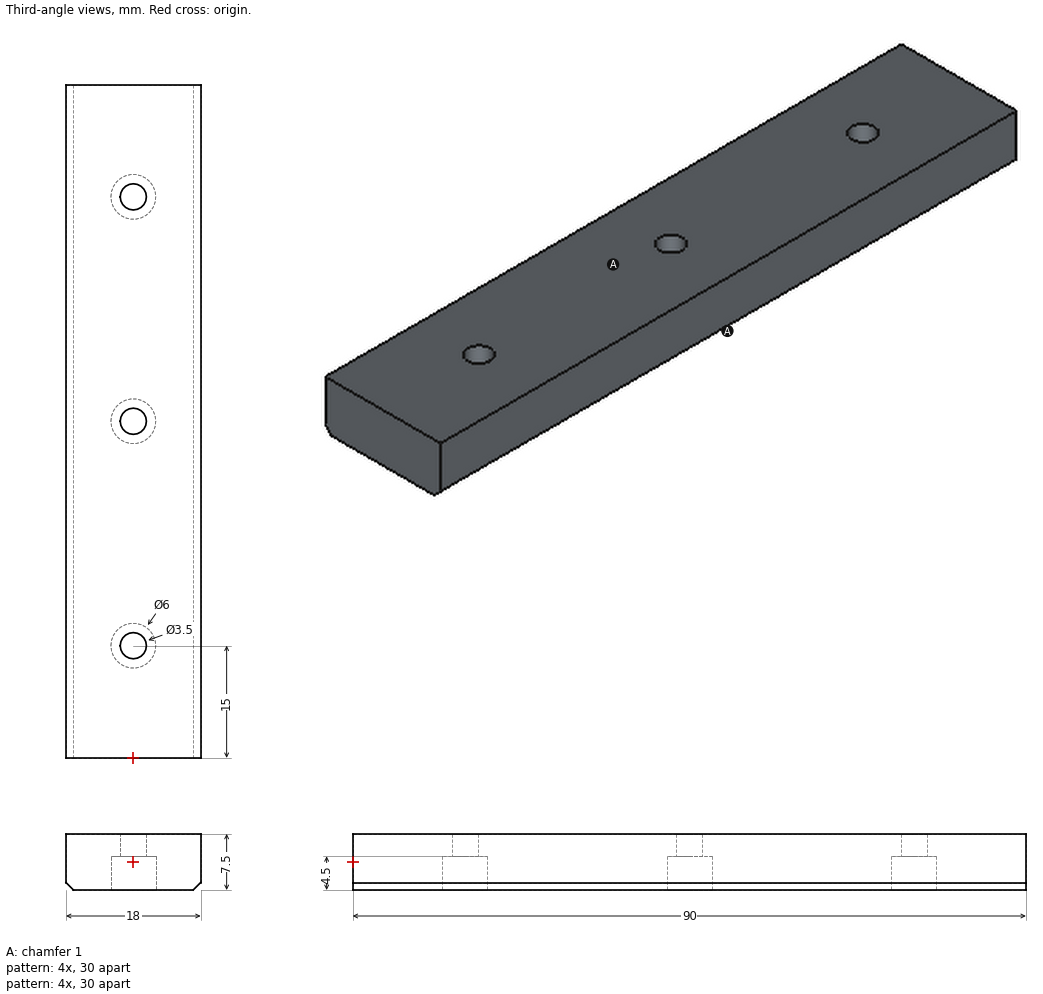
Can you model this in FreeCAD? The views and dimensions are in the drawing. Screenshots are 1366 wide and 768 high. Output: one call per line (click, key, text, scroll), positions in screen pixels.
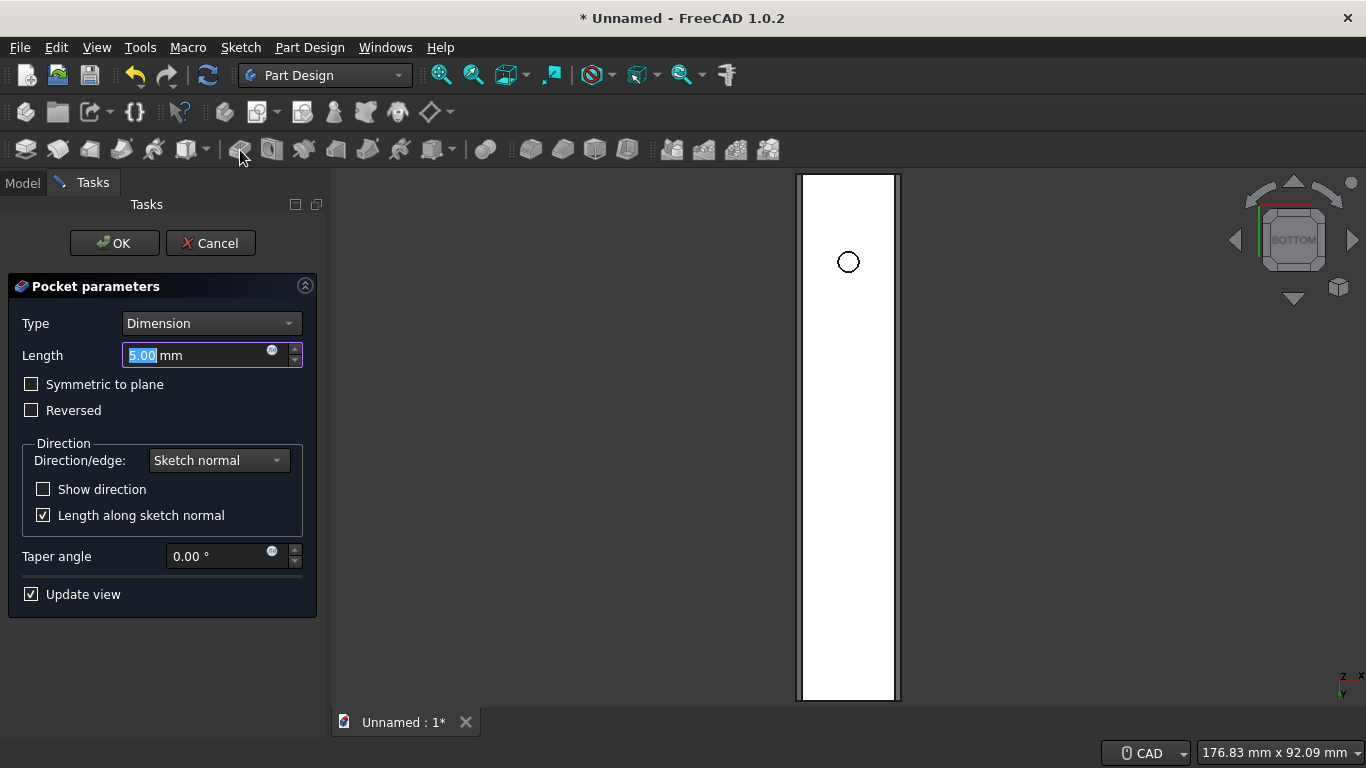
click(212, 324)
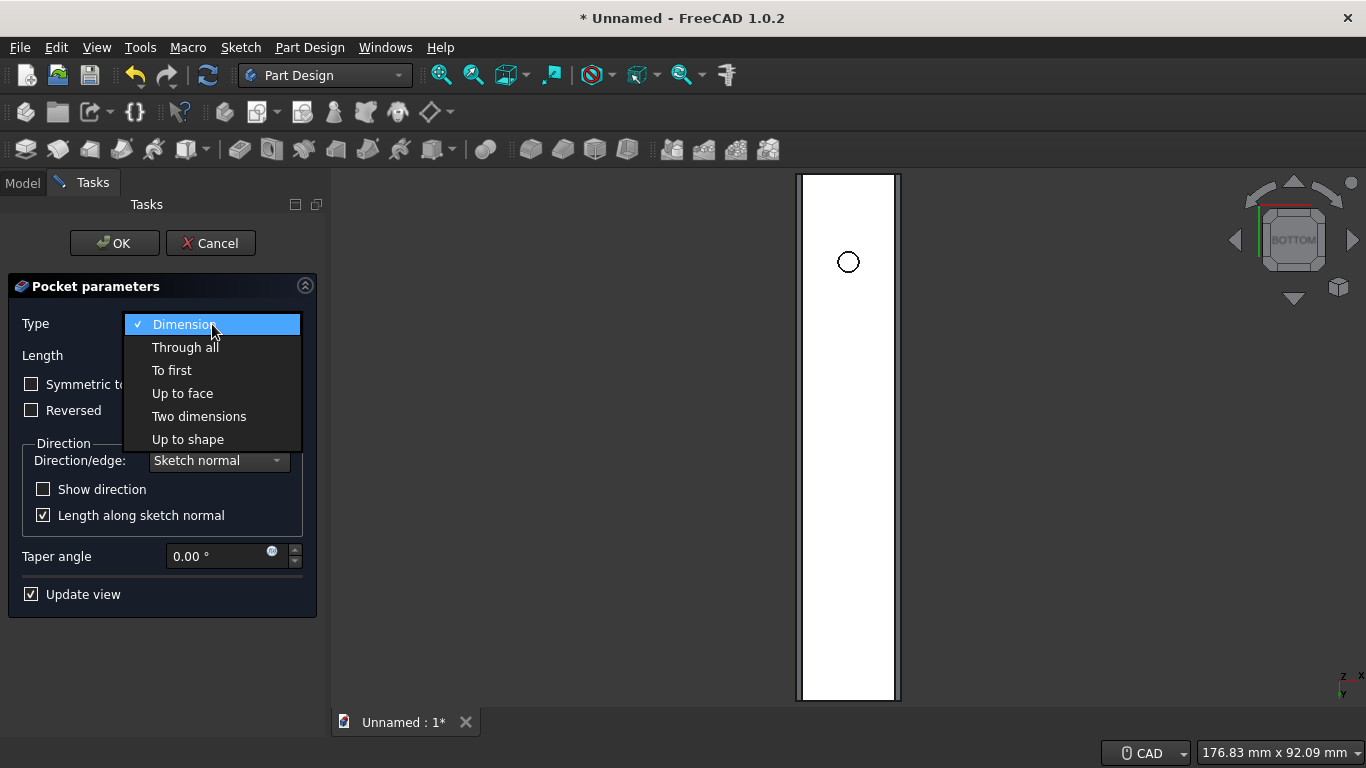
click(212, 348)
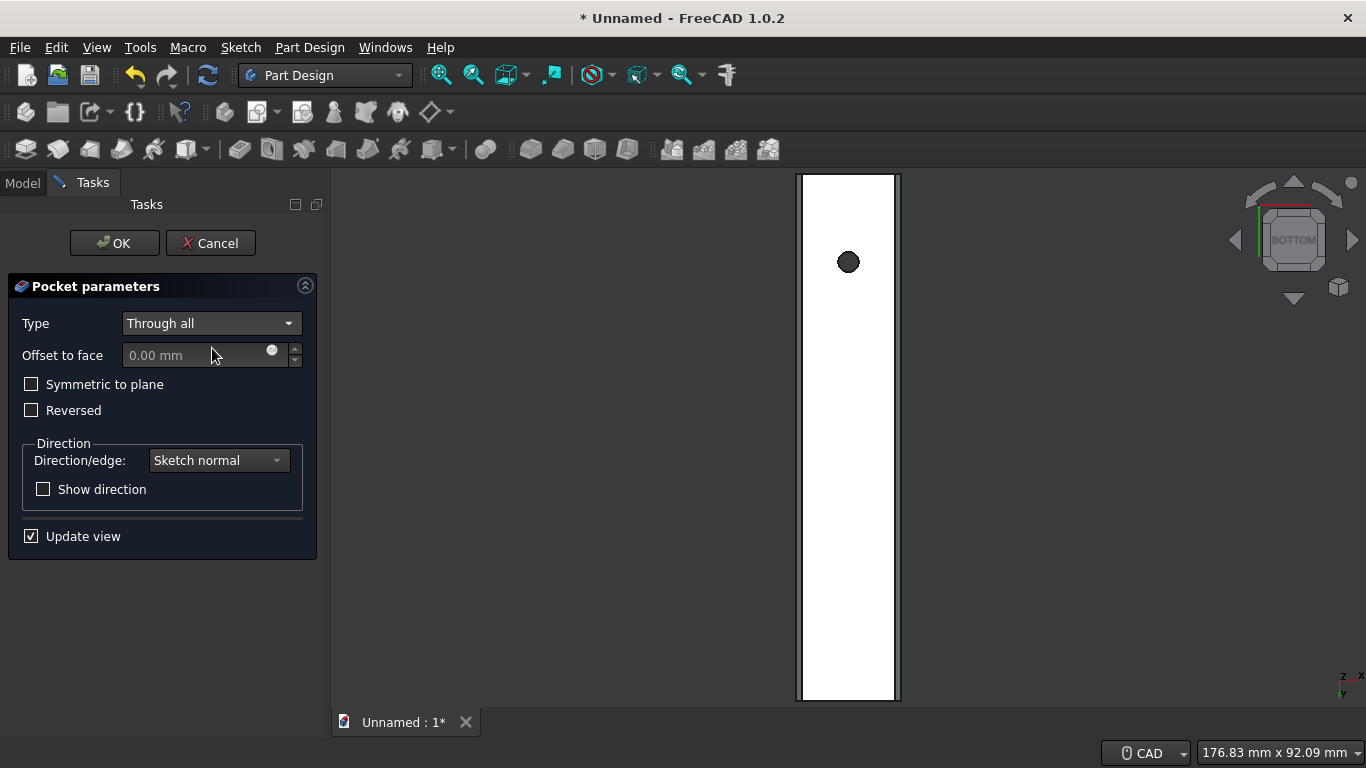
click(115, 243)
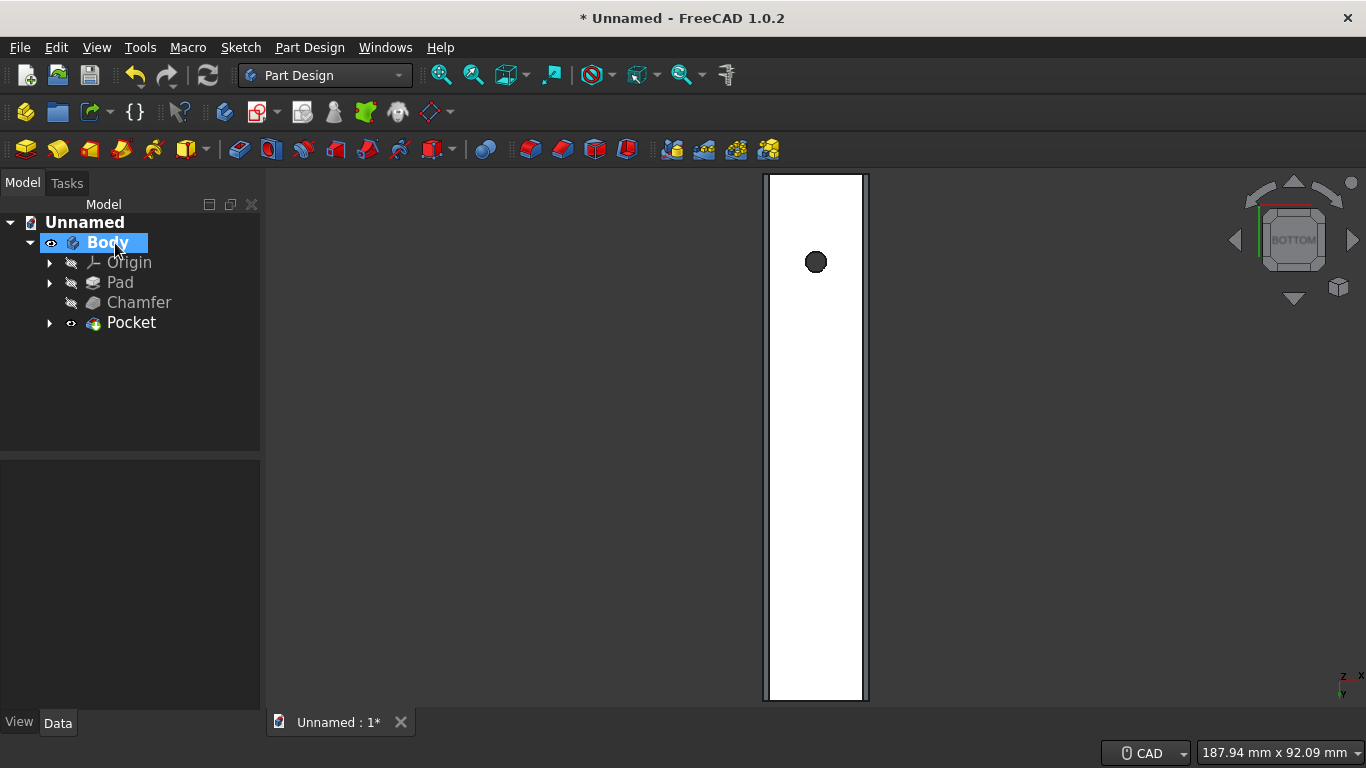
click(816, 587)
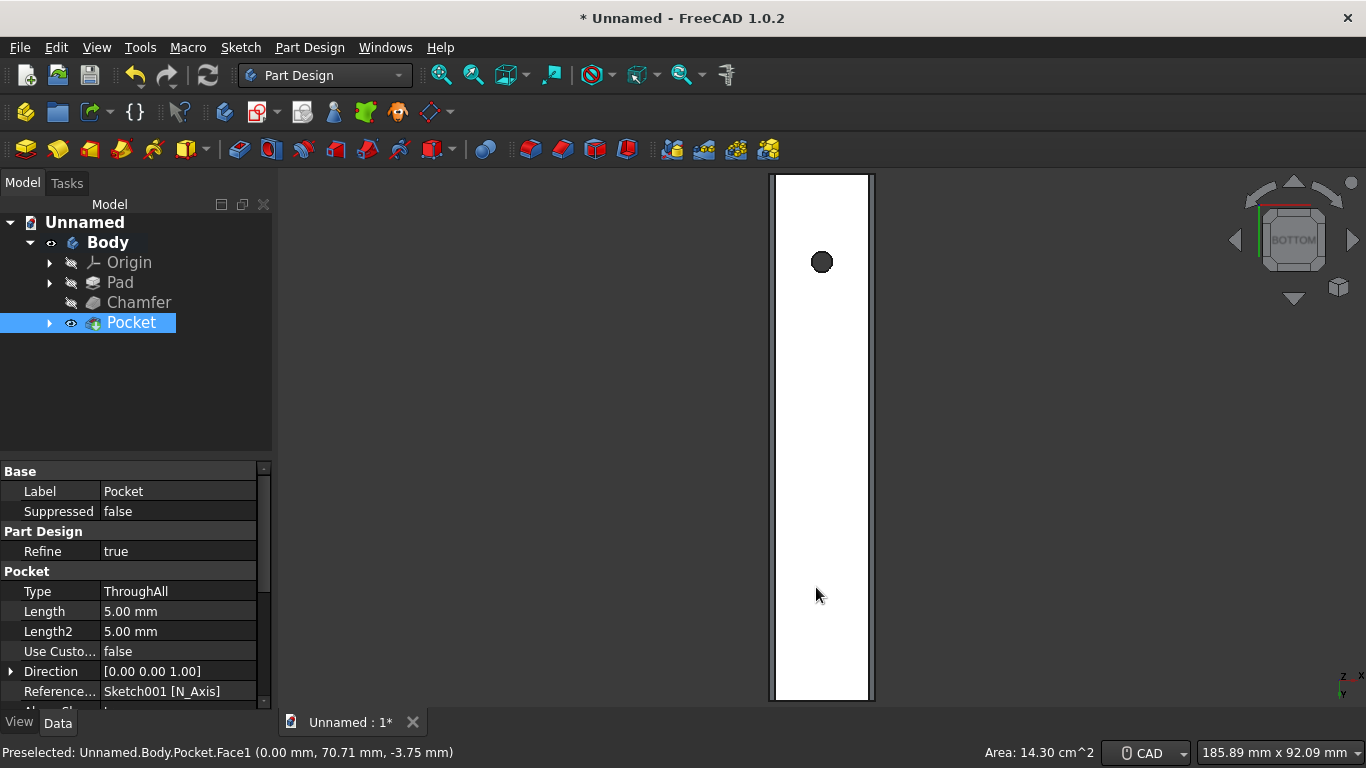
click(258, 112)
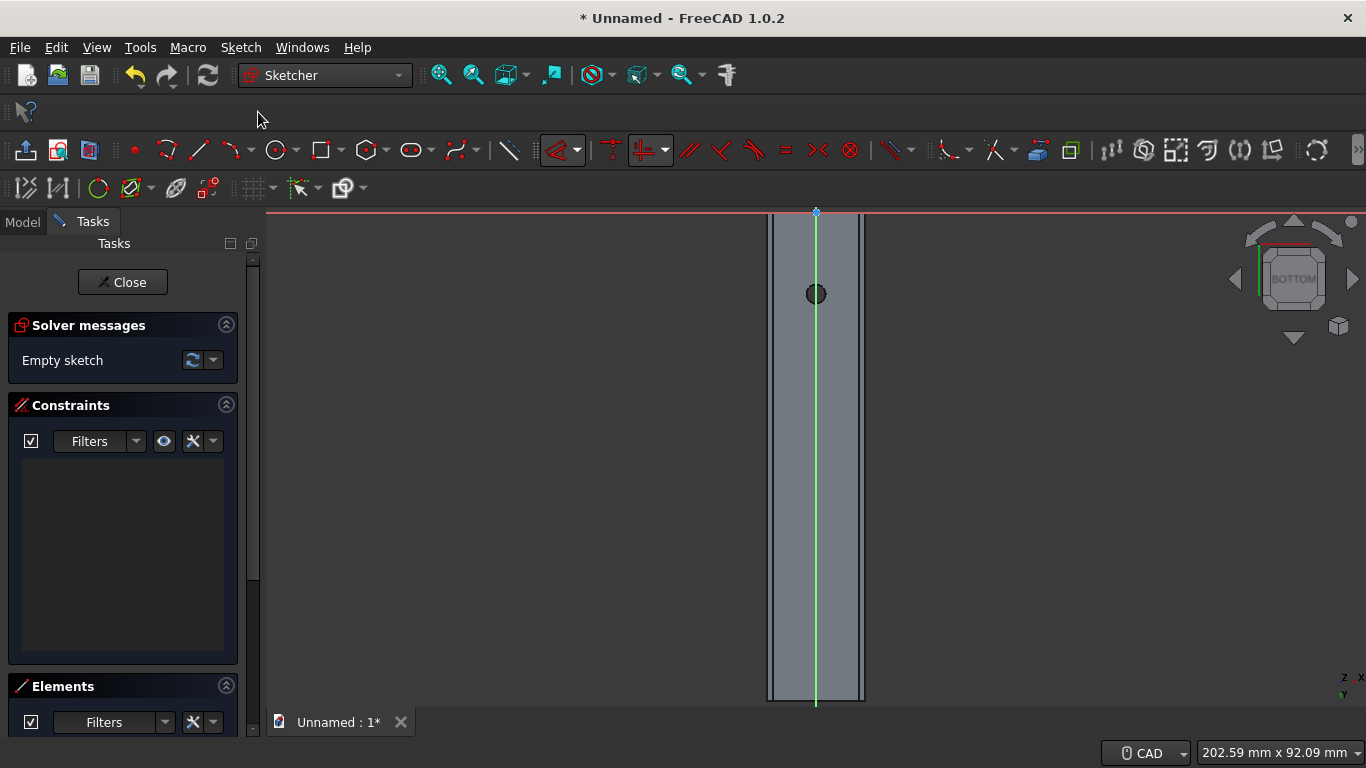
scroll(825, 274, up, 11)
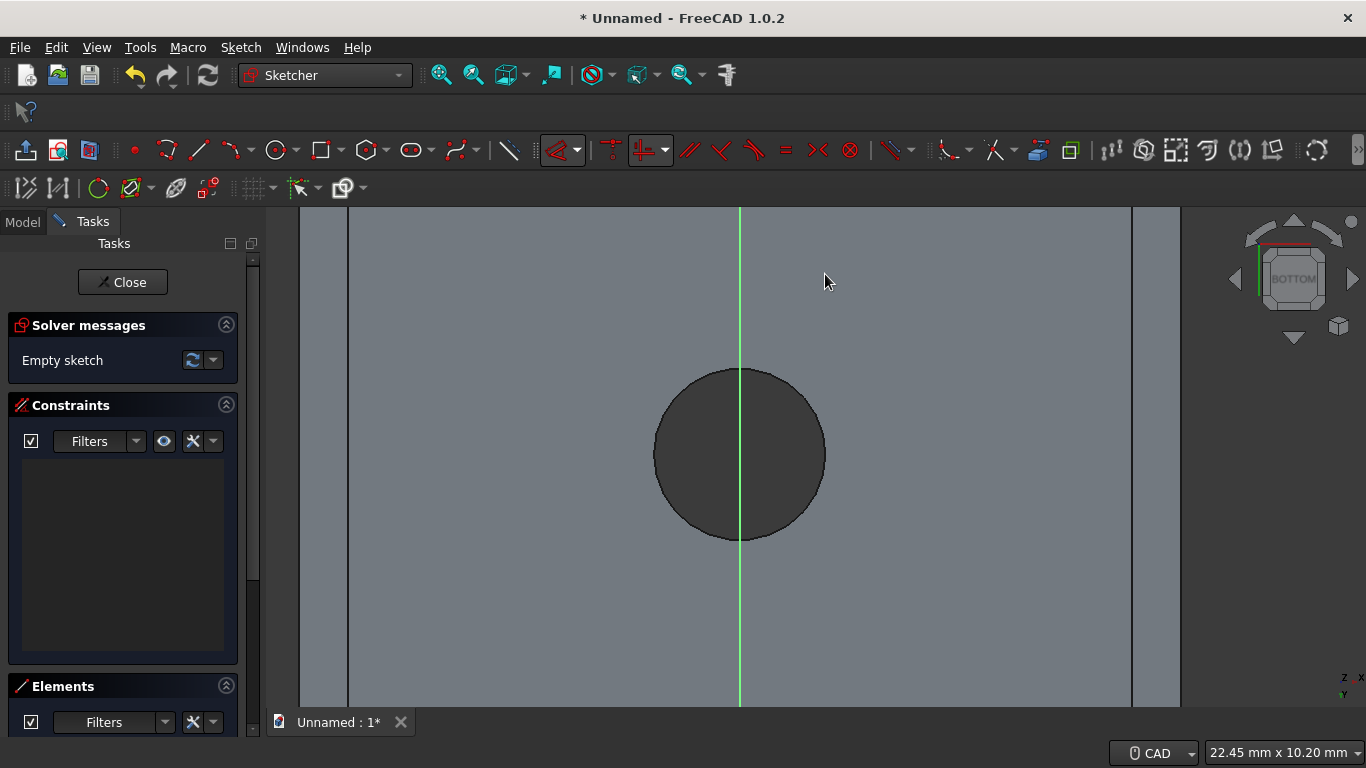
click(276, 150)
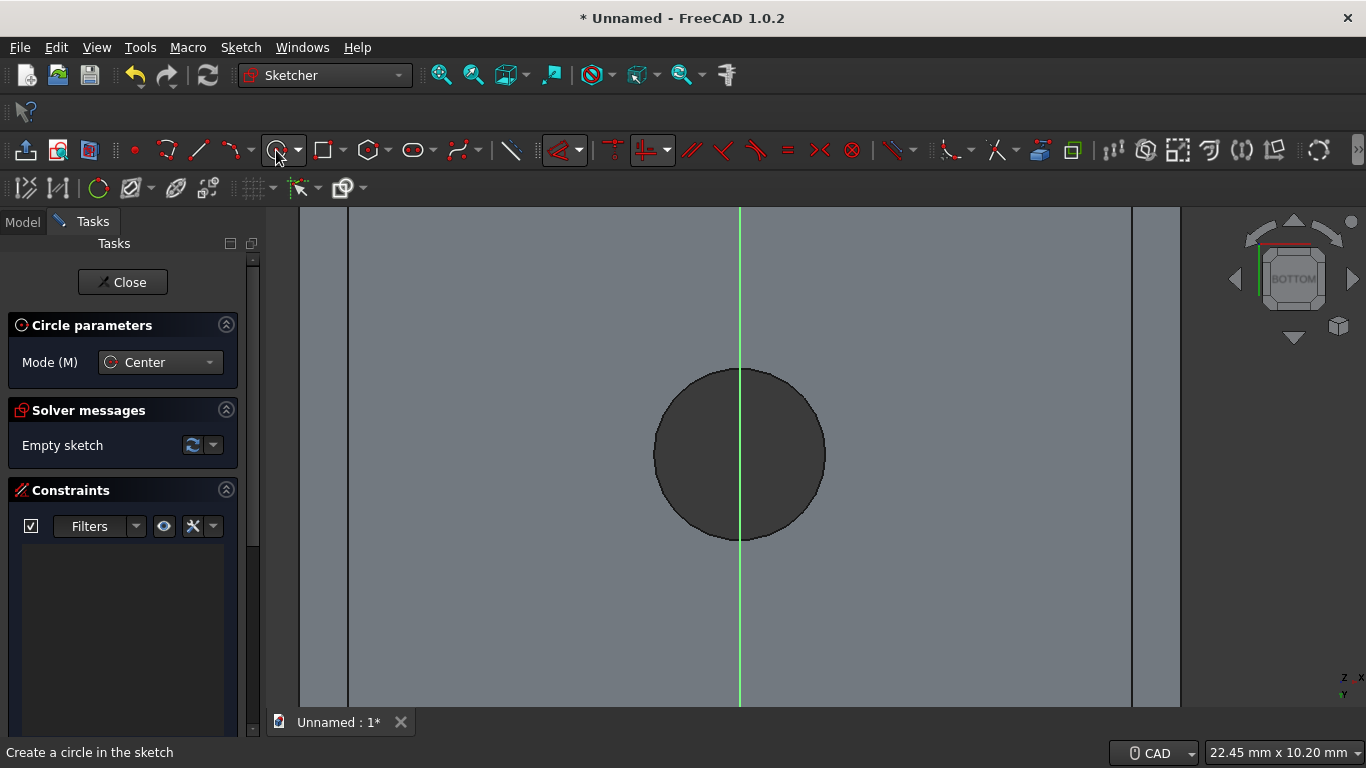
click(740, 454)
click(844, 350)
key(Escape)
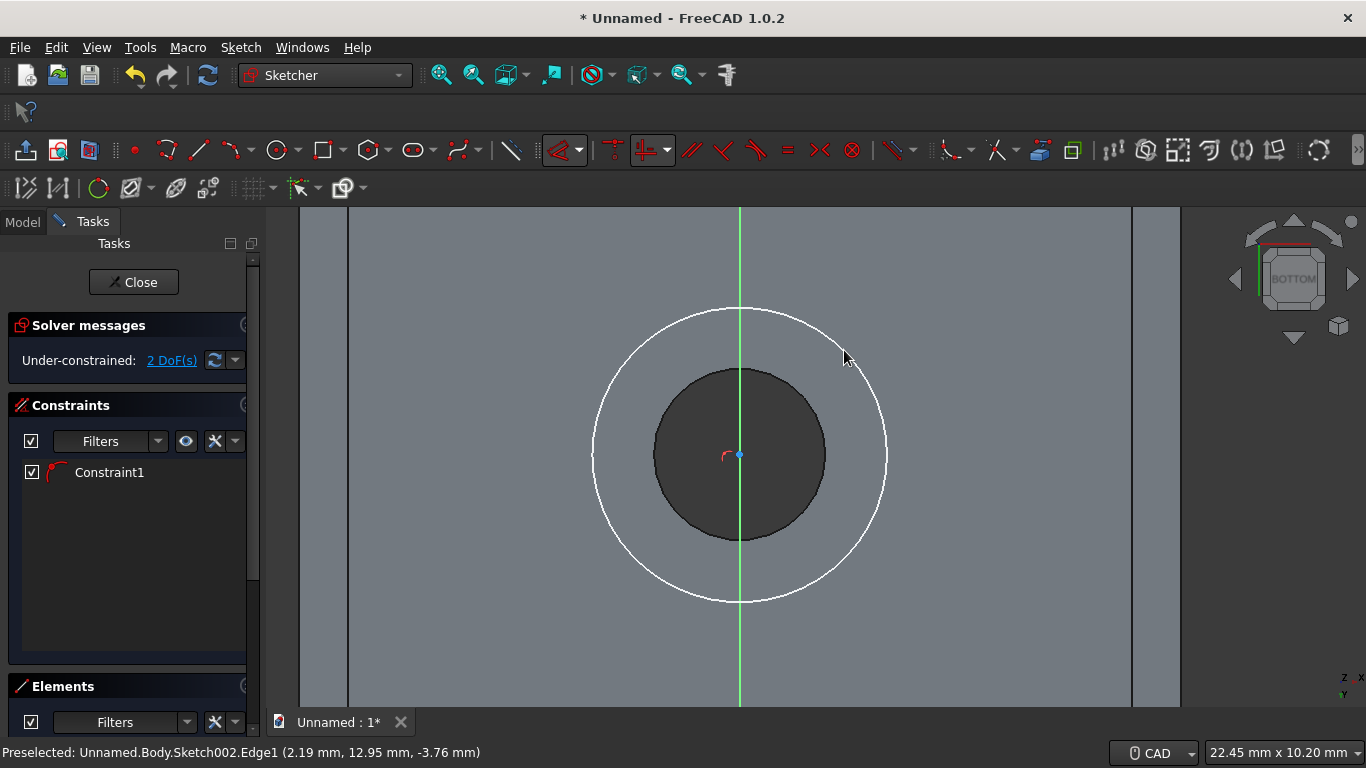
click(844, 351)